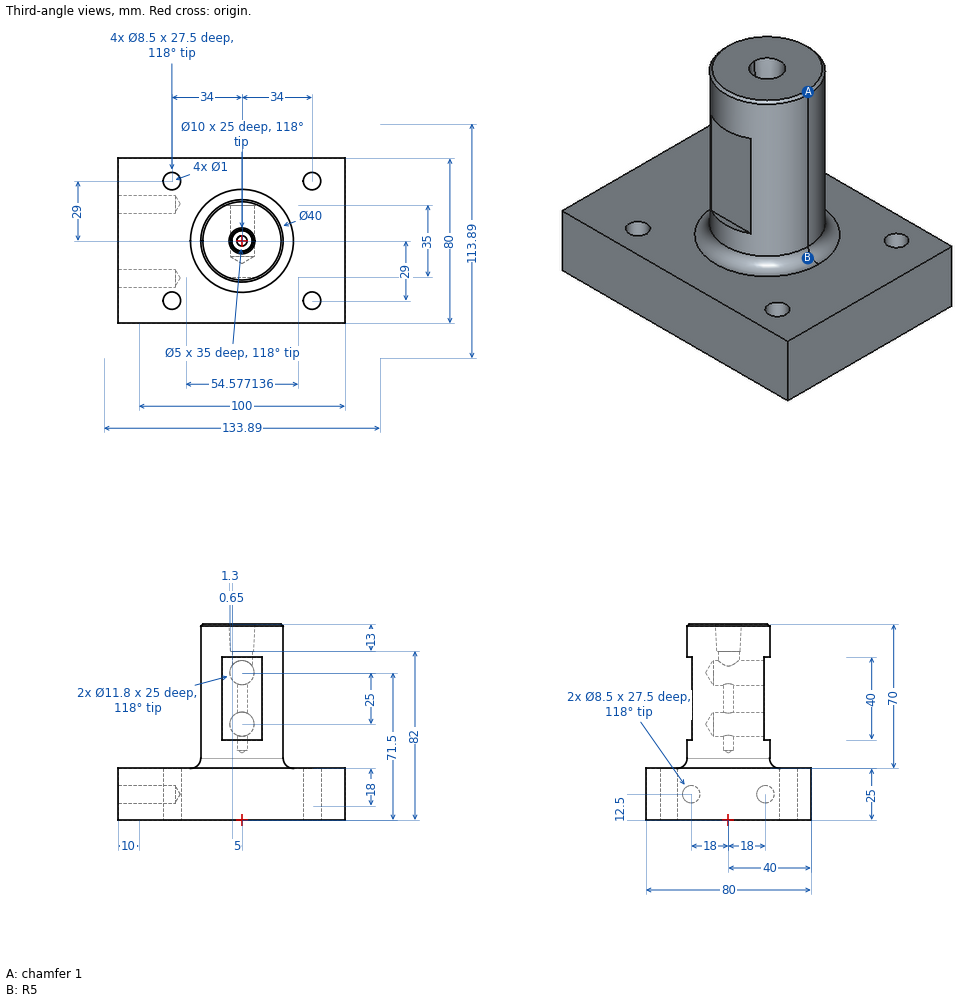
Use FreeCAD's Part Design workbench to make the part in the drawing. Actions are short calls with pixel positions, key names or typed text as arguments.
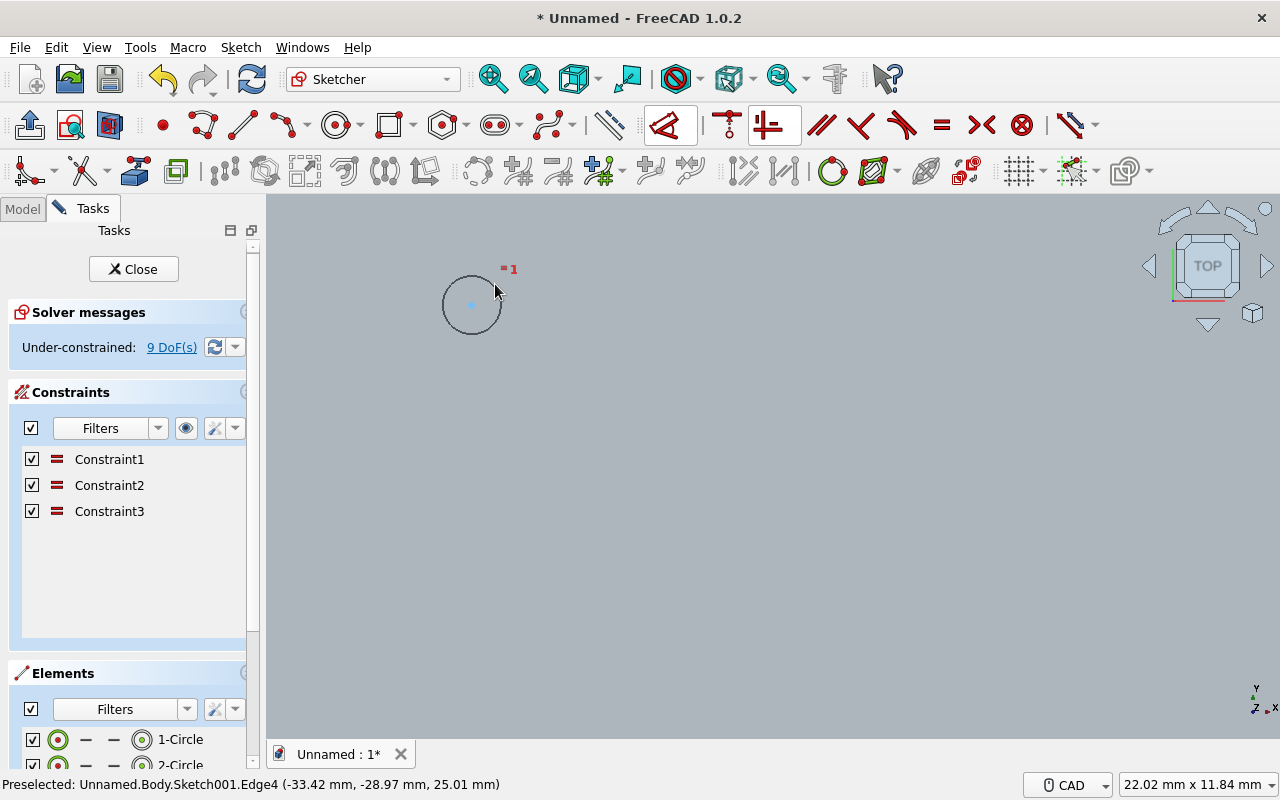
click(492, 285)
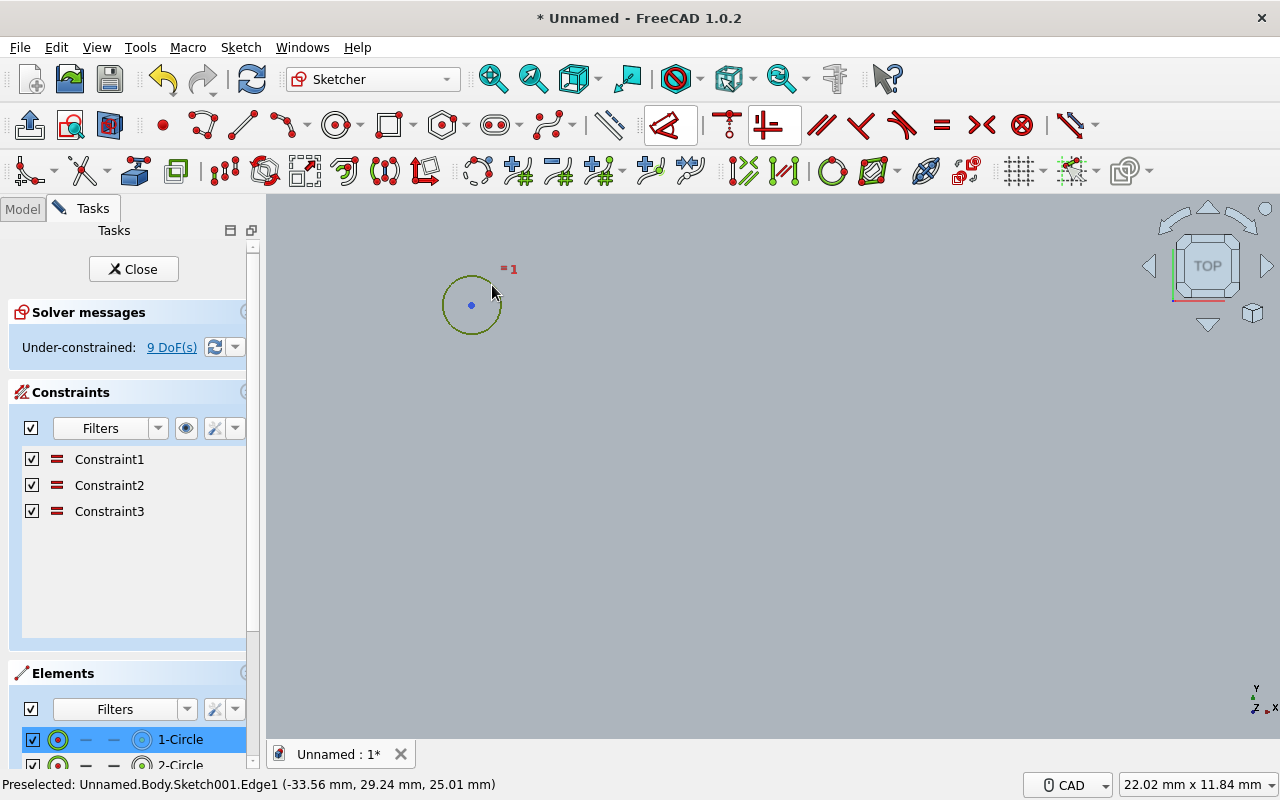
key(k)
key(o)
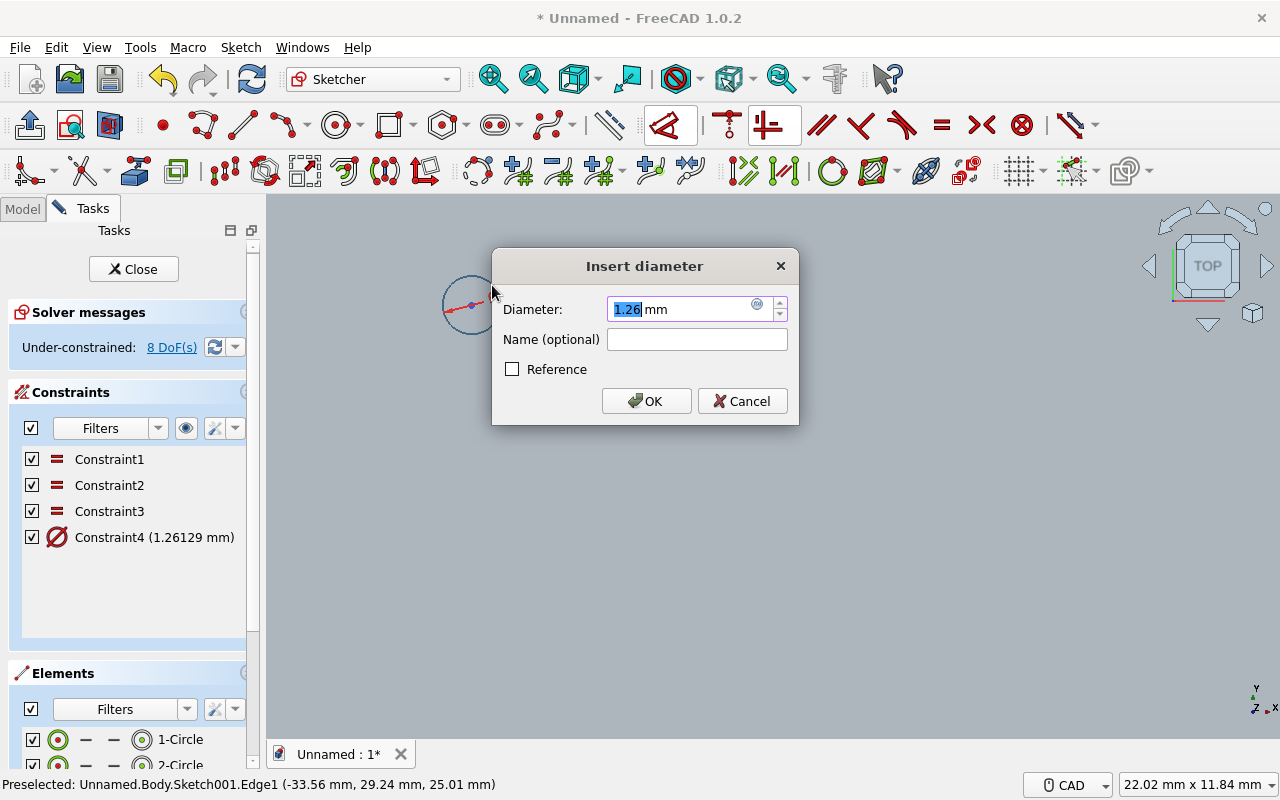
text(1)
key(Return)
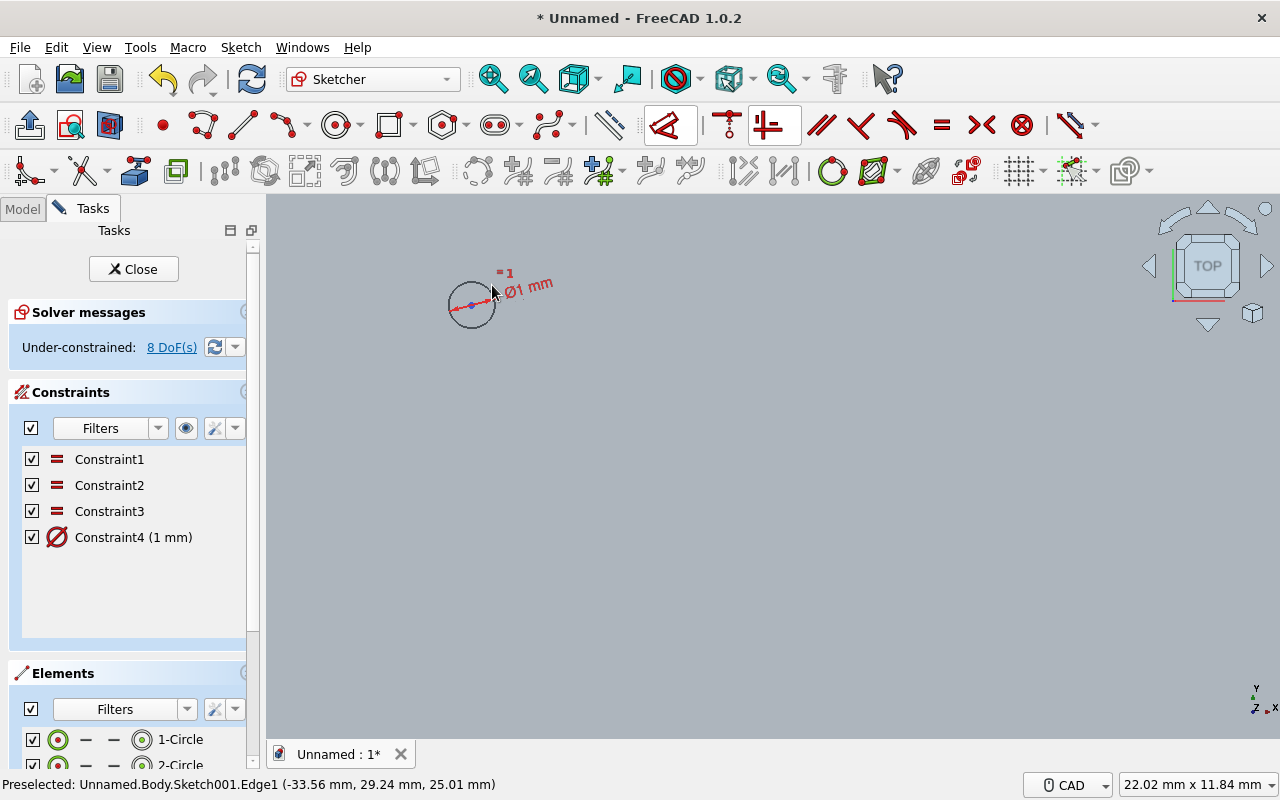
scroll(495, 284, down, 10)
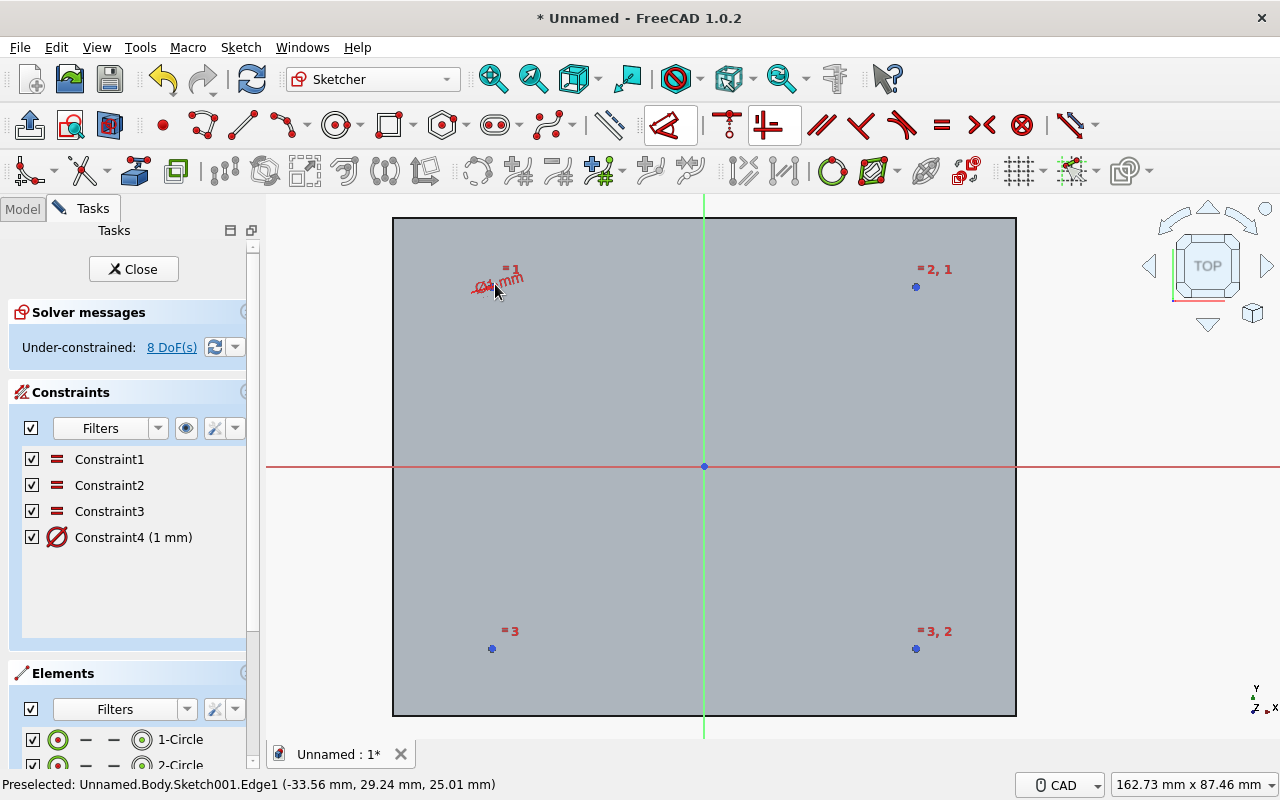
click(492, 287)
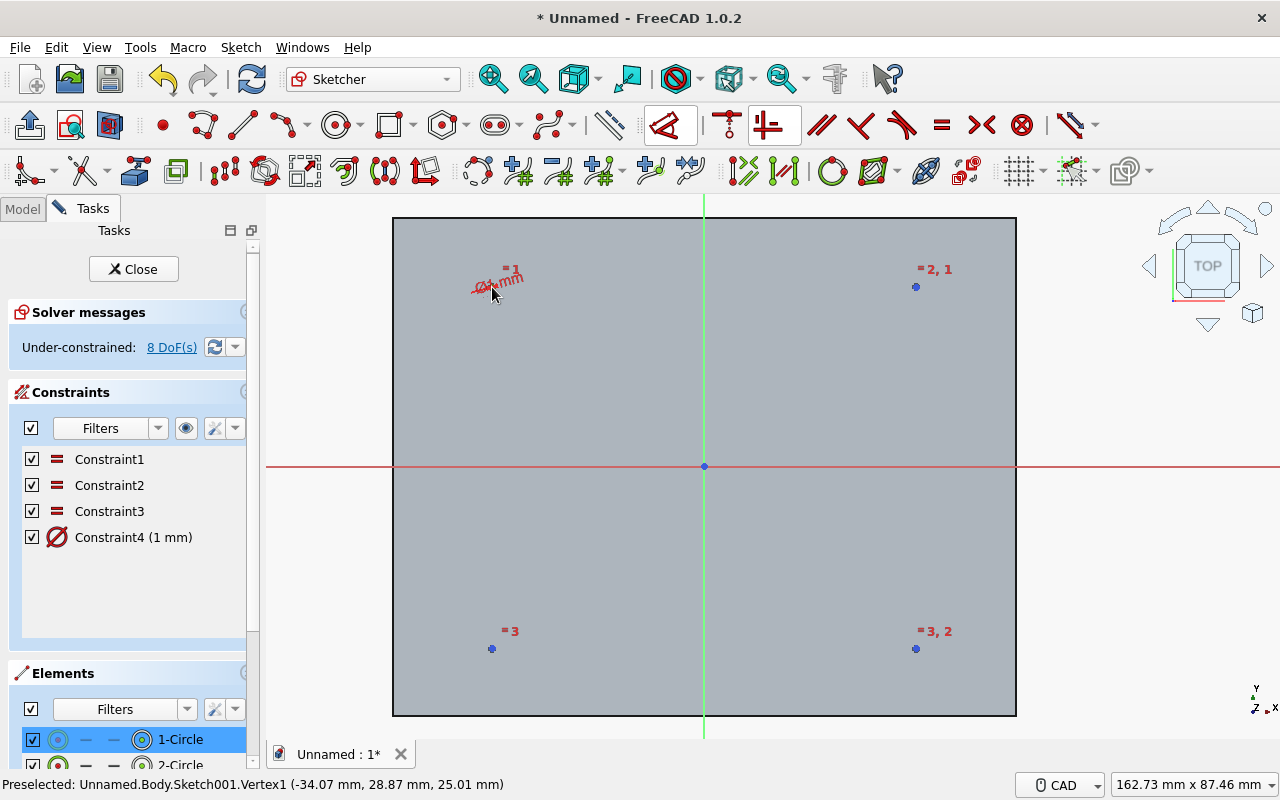
key(l)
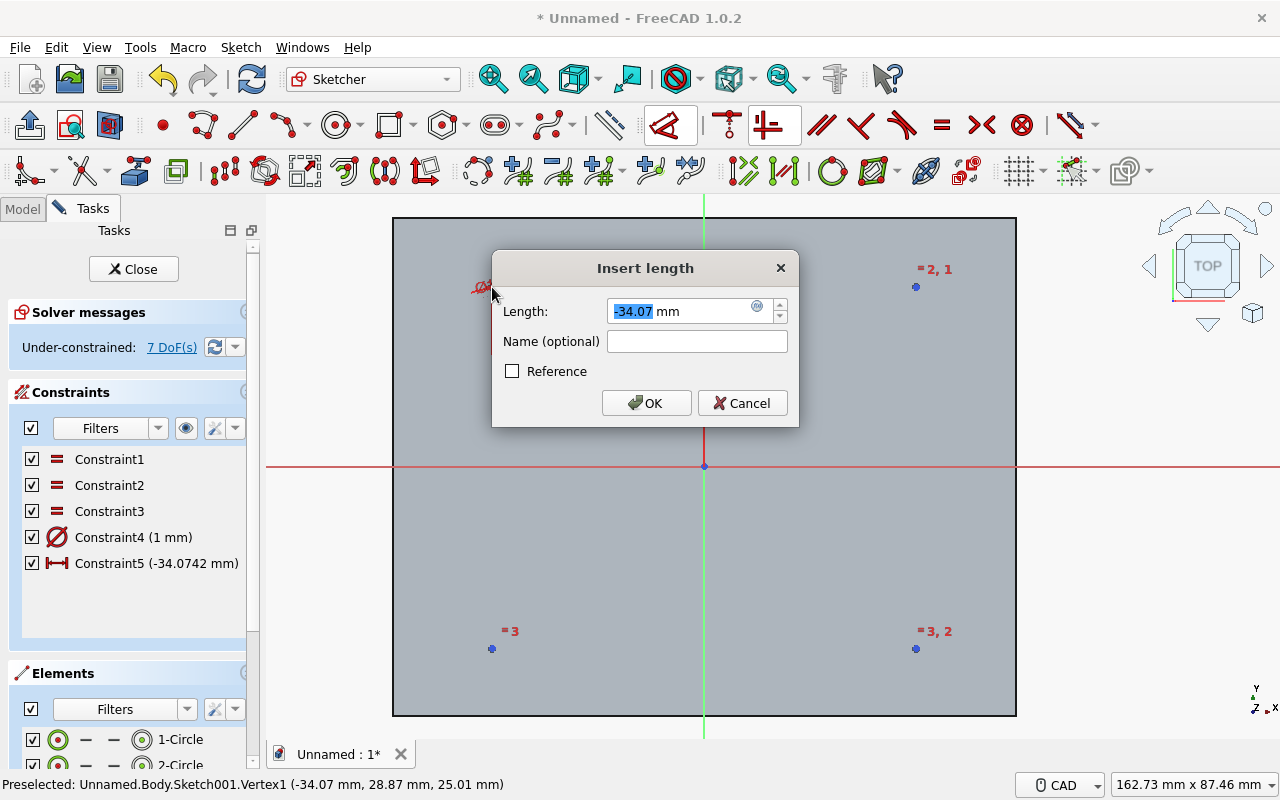
text(-34)
key(Return)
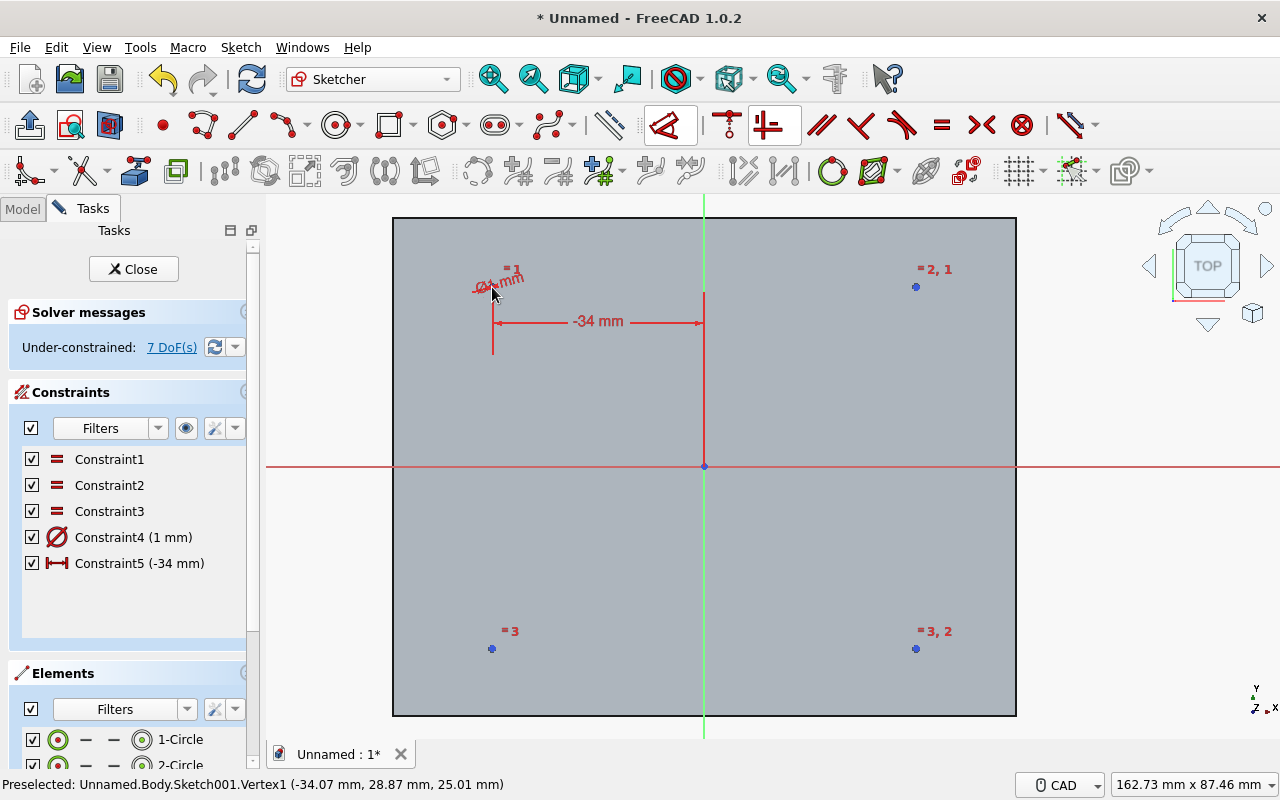
click(493, 287)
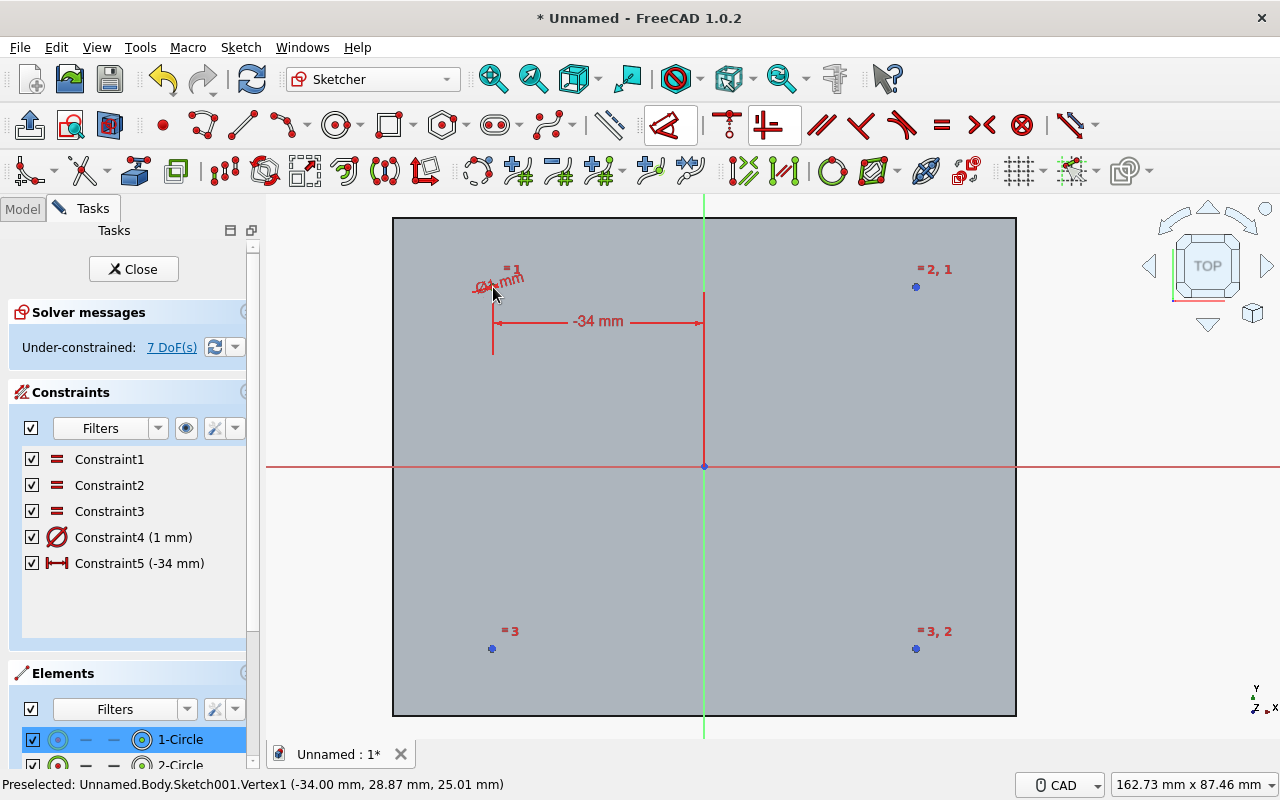
key(i)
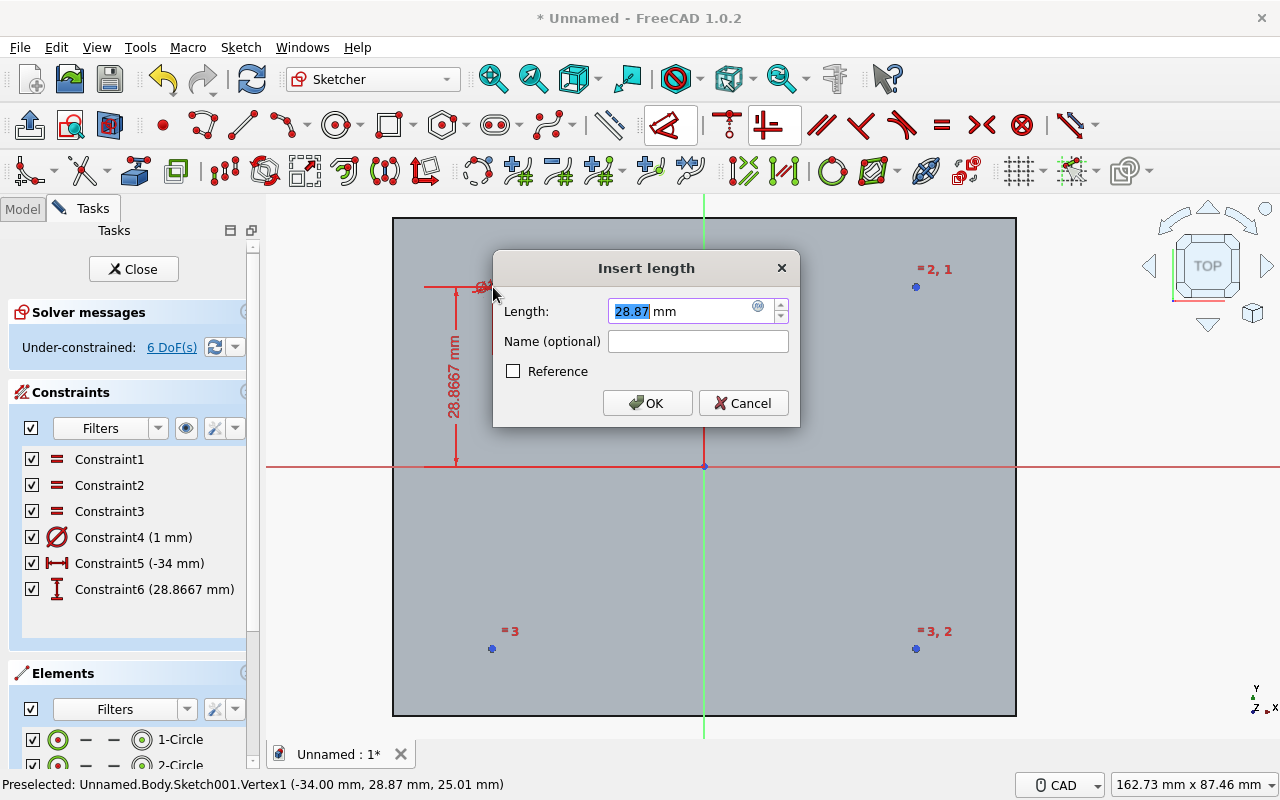
text(29)
key(Return)